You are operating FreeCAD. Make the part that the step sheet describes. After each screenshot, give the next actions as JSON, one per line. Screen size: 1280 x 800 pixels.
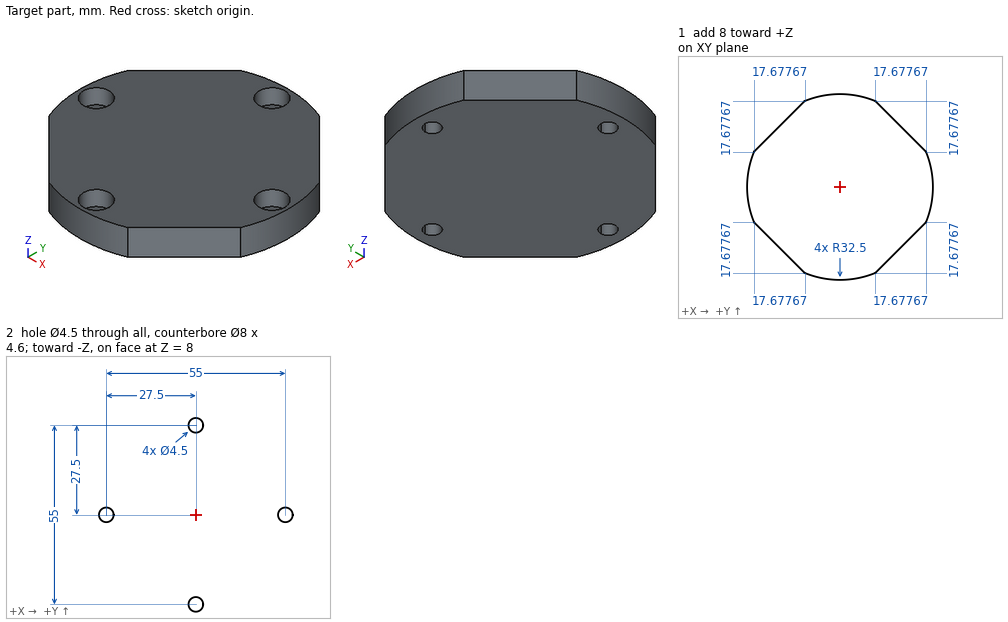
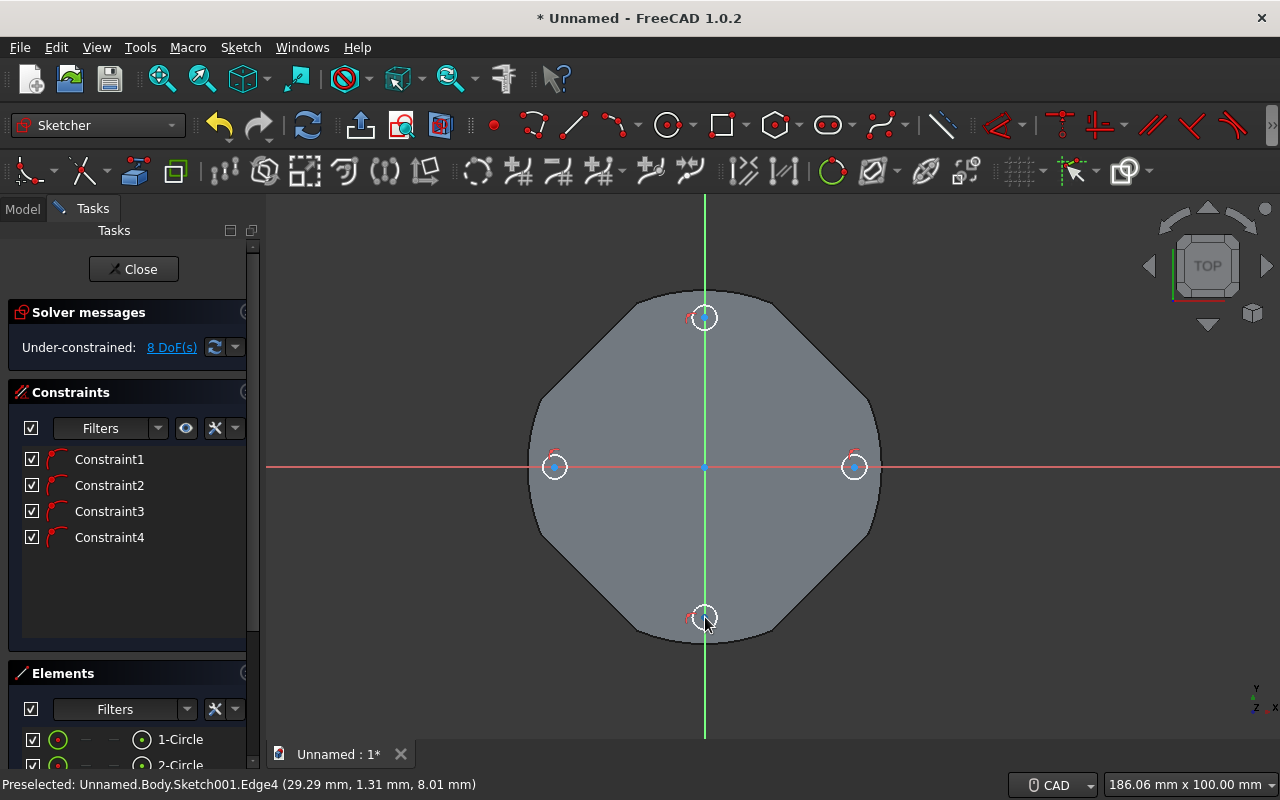
{"action": "scroll", "coordinate": [713, 309], "scroll_direction": "up", "scroll_amount": 3}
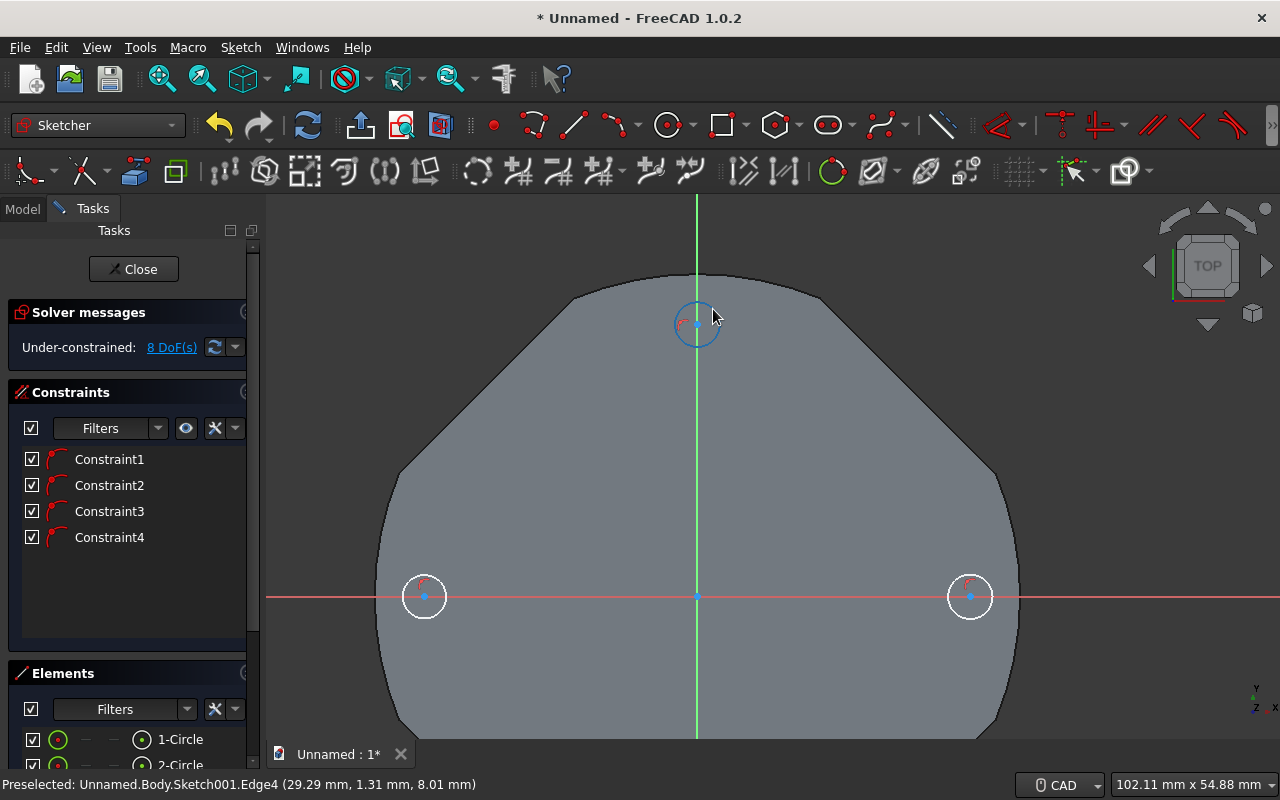
{"action": "left_click", "coordinate": [713, 309]}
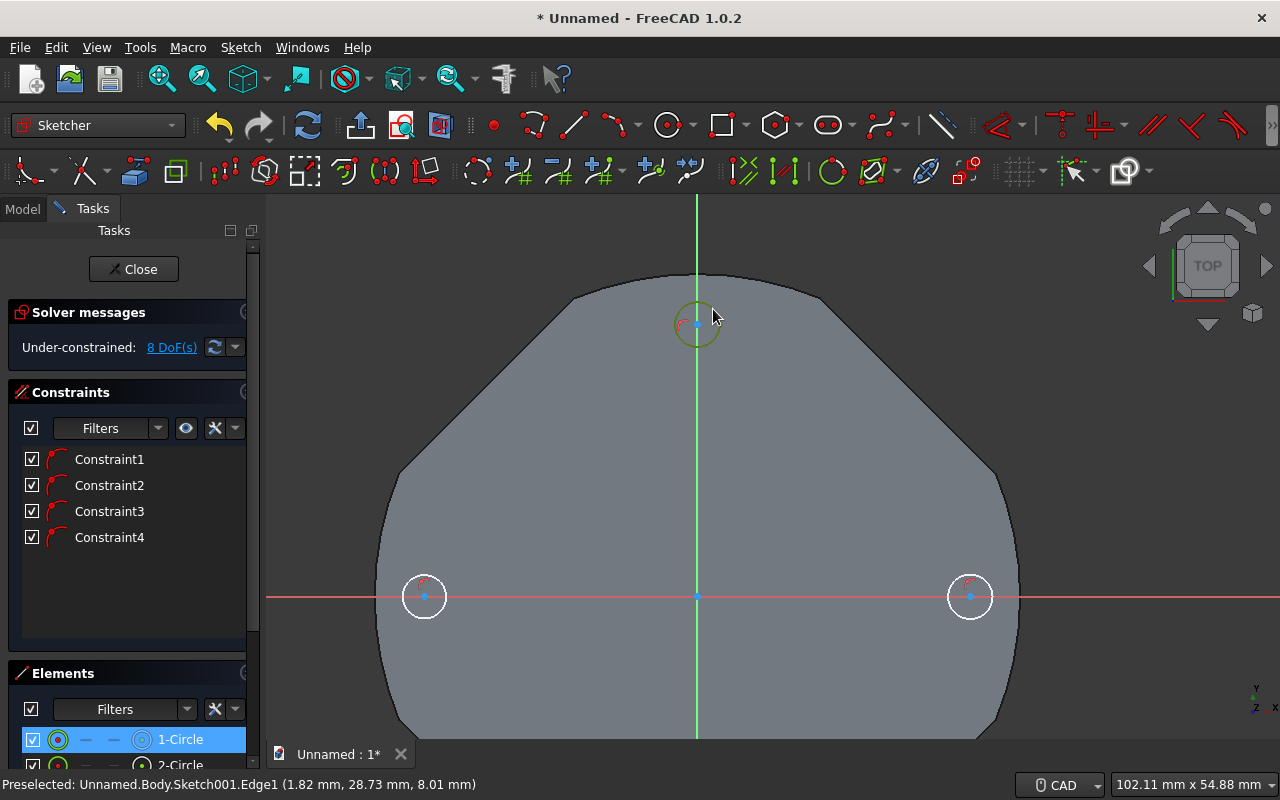
{"action": "left_click", "coordinate": [440, 581]}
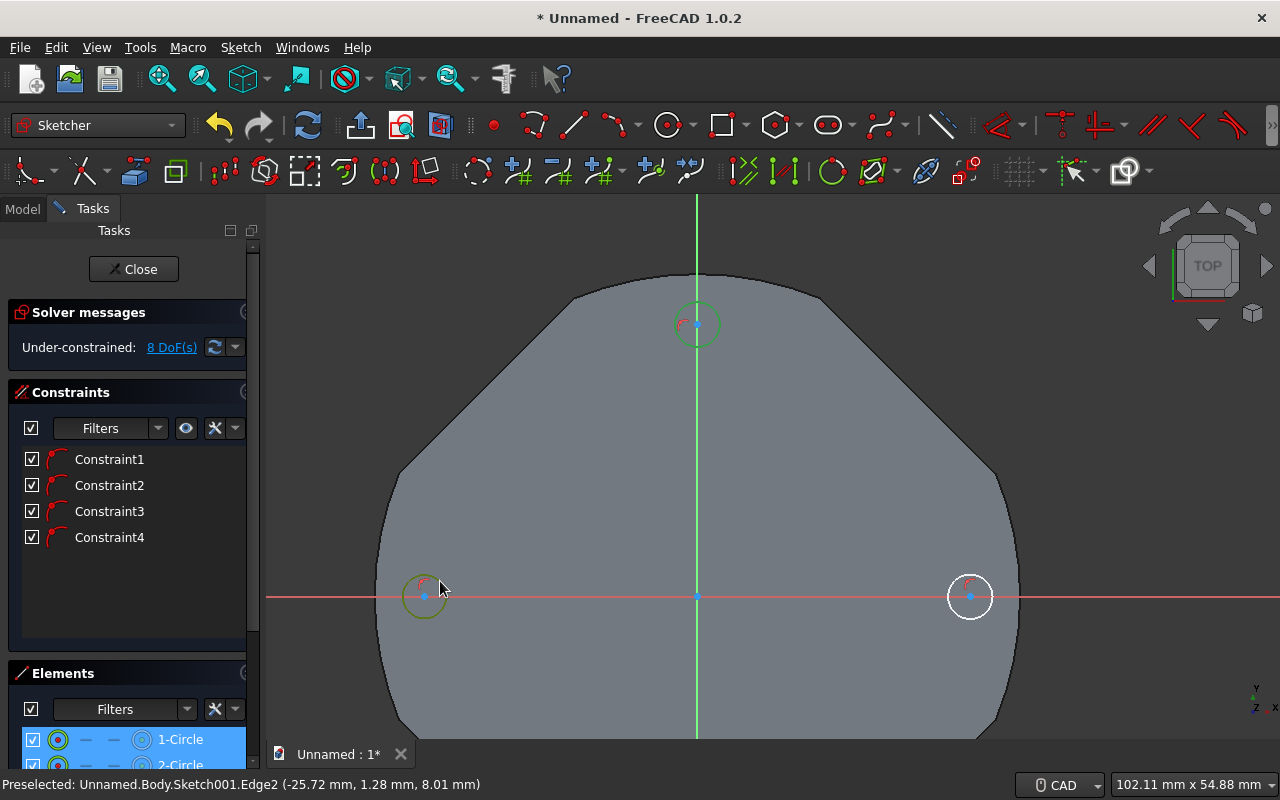
{"action": "scroll", "coordinate": [713, 308], "scroll_direction": "down", "scroll_amount": 3}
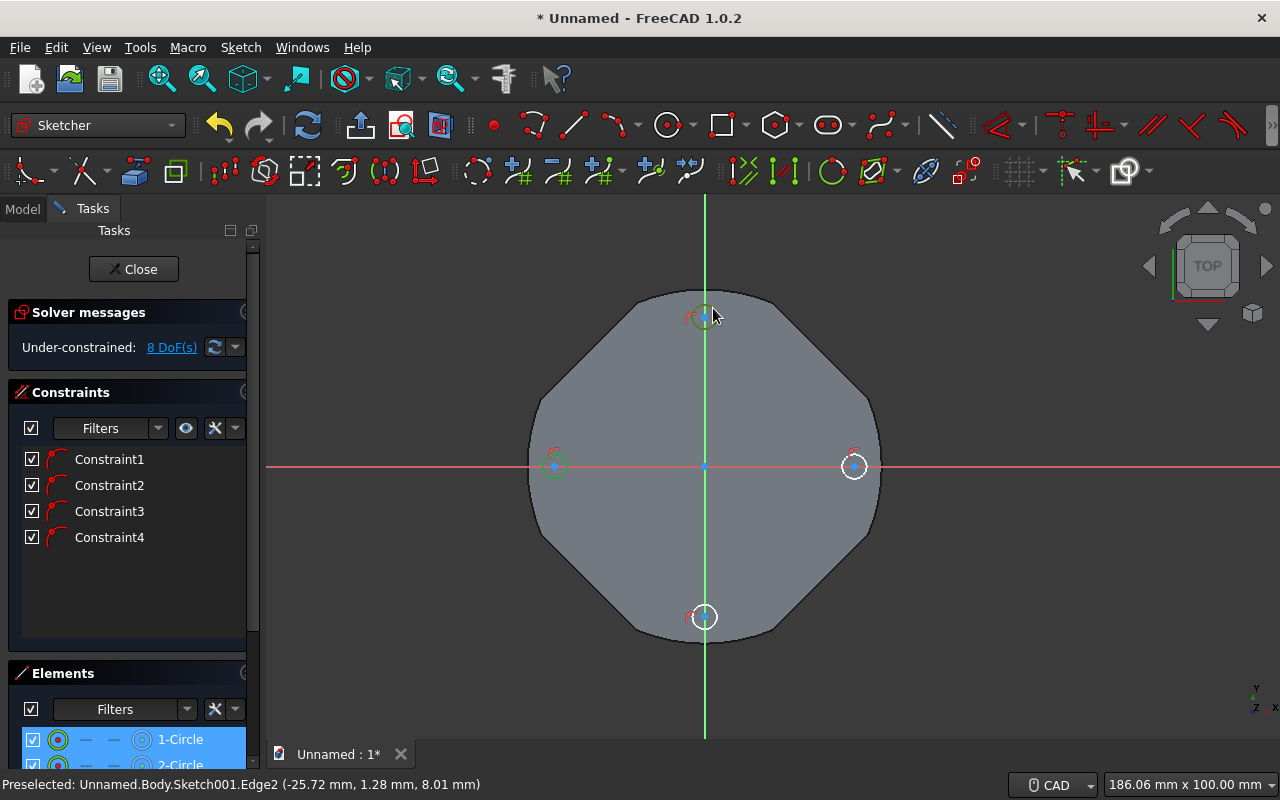
{"action": "scroll", "coordinate": [713, 608], "scroll_direction": "up", "scroll_amount": 3}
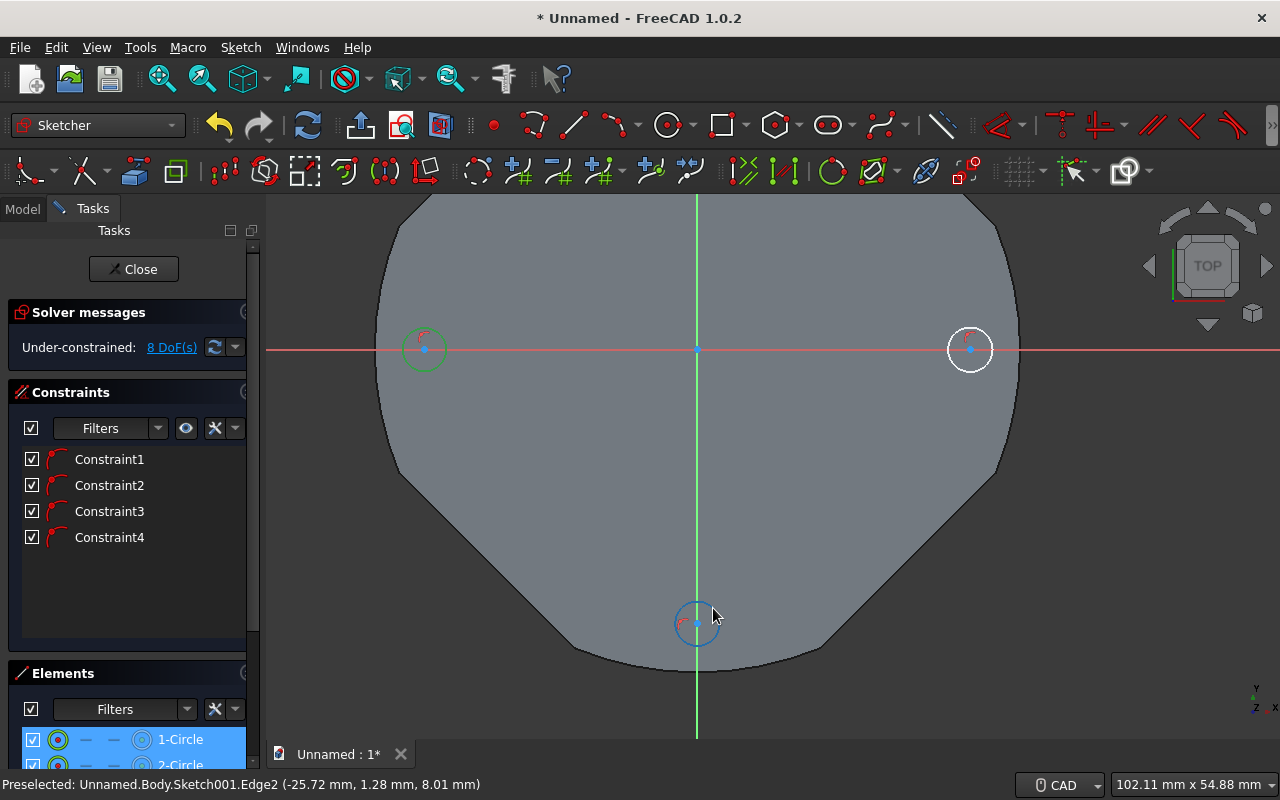
{"action": "left_click", "coordinate": [713, 608]}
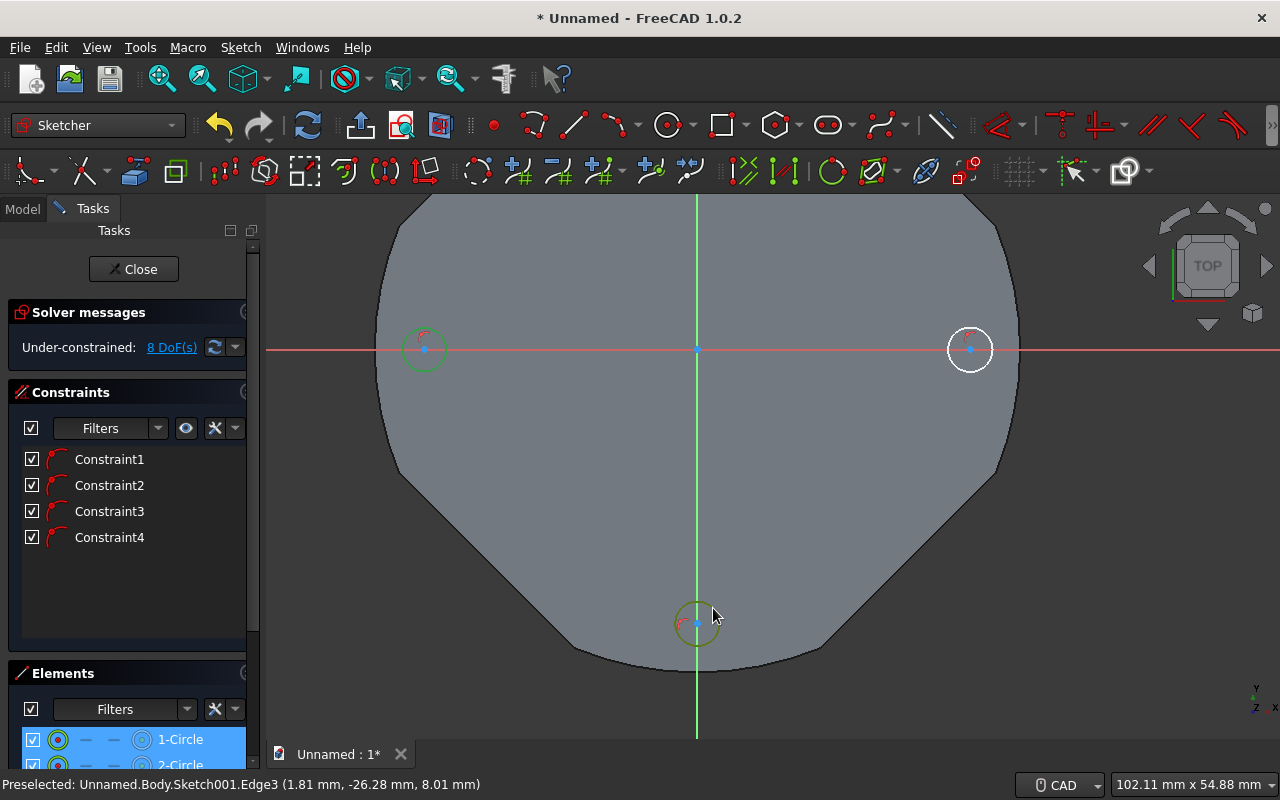
{"action": "left_click", "coordinate": [986, 334]}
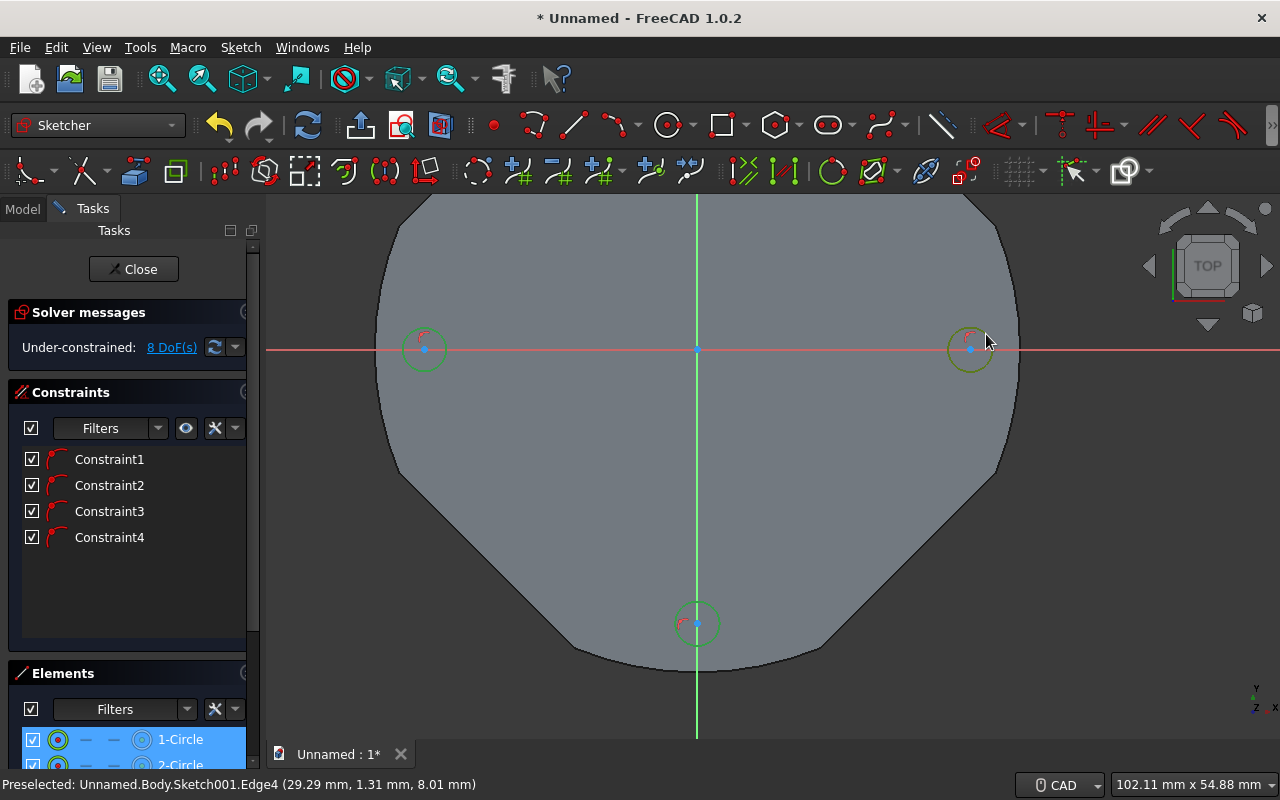
{"action": "key", "text": "e"}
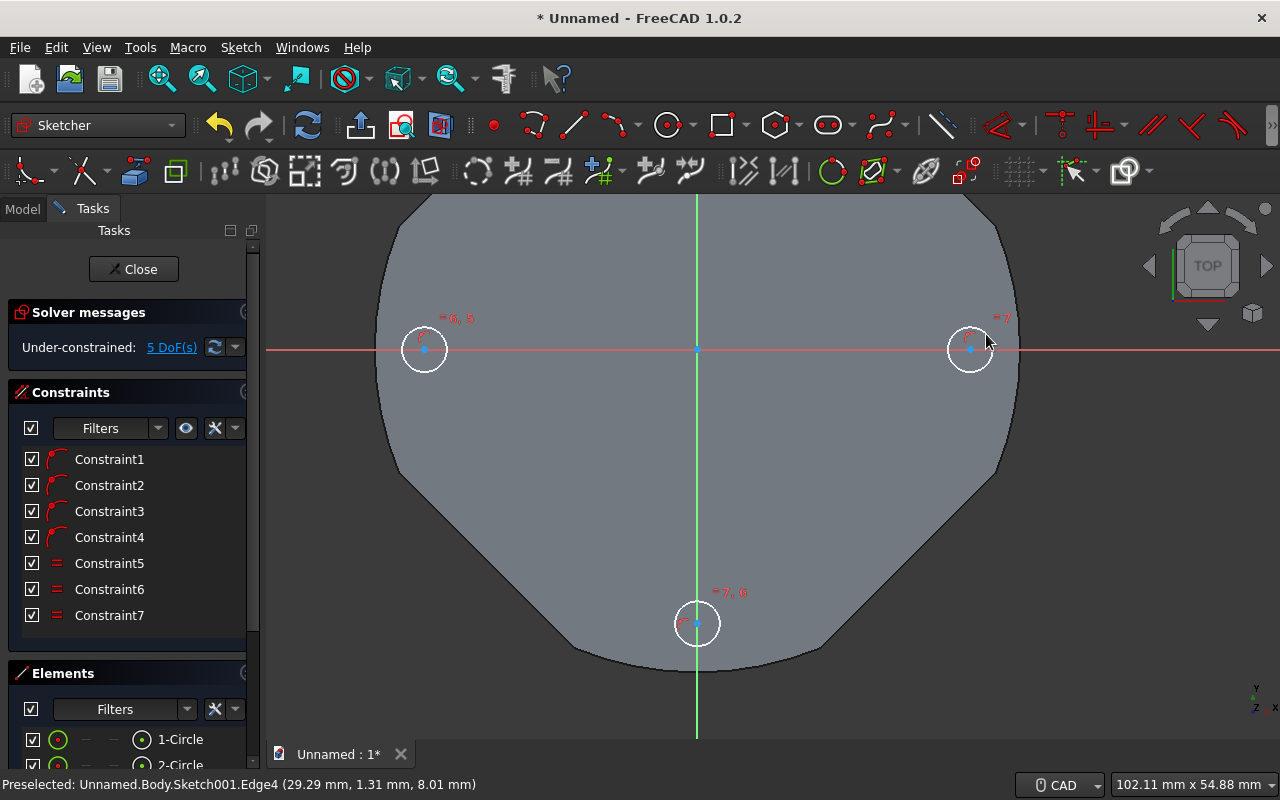
{"action": "left_click", "coordinate": [998, 126]}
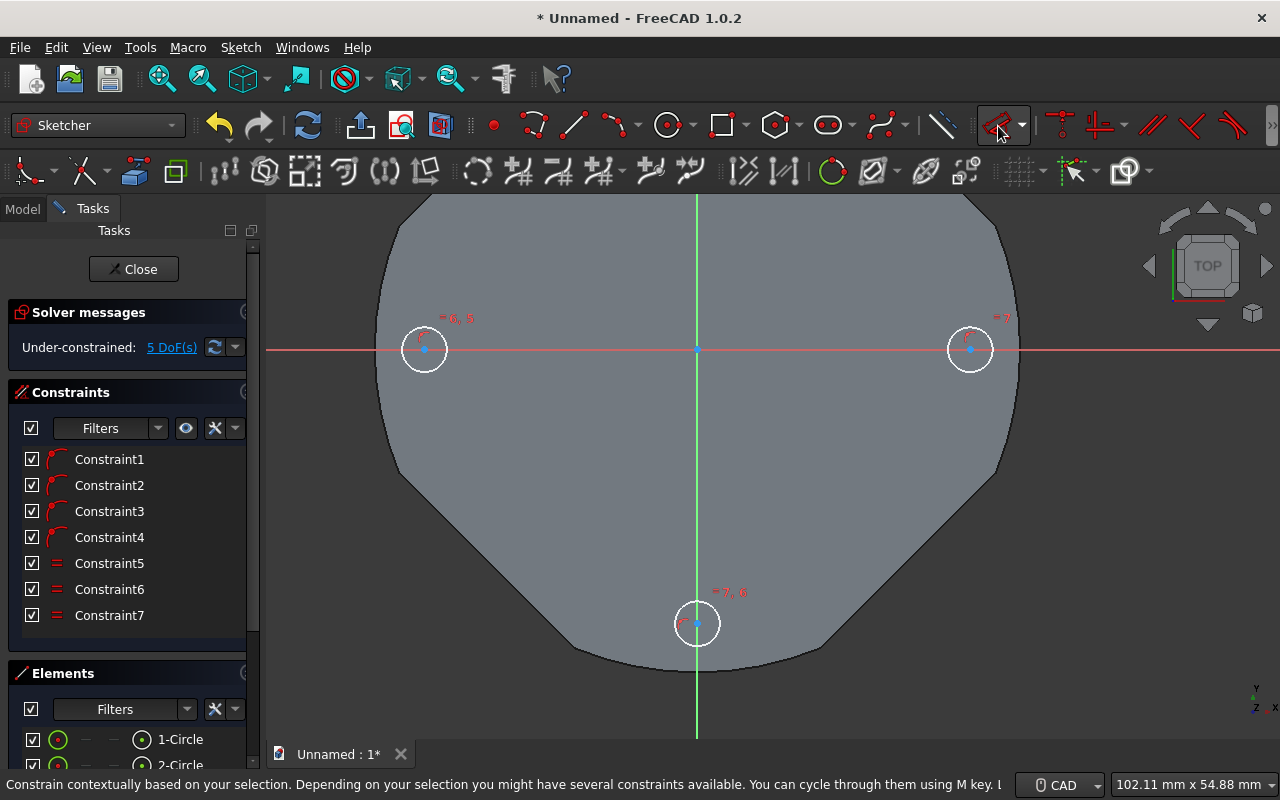
{"action": "scroll", "coordinate": [713, 609], "scroll_direction": "down", "scroll_amount": 3}